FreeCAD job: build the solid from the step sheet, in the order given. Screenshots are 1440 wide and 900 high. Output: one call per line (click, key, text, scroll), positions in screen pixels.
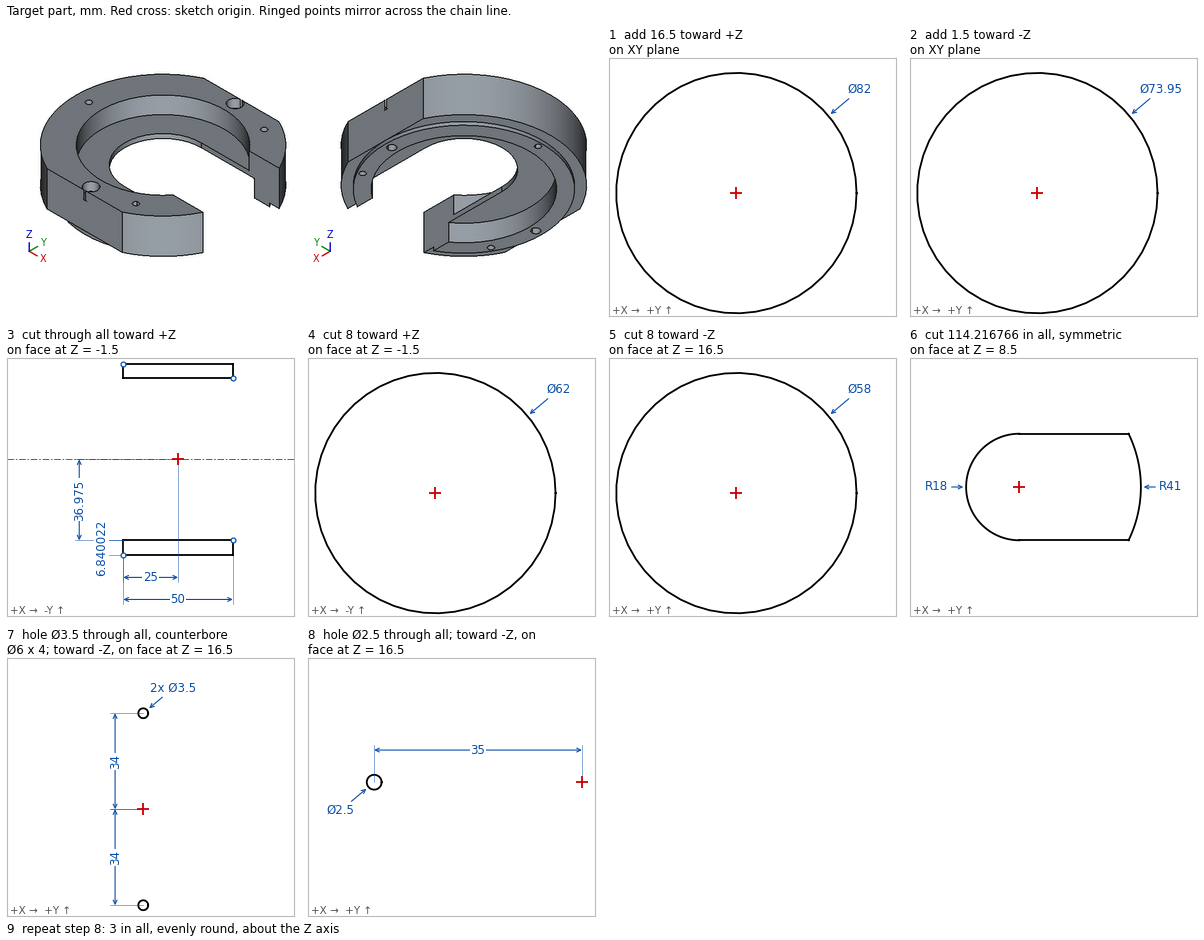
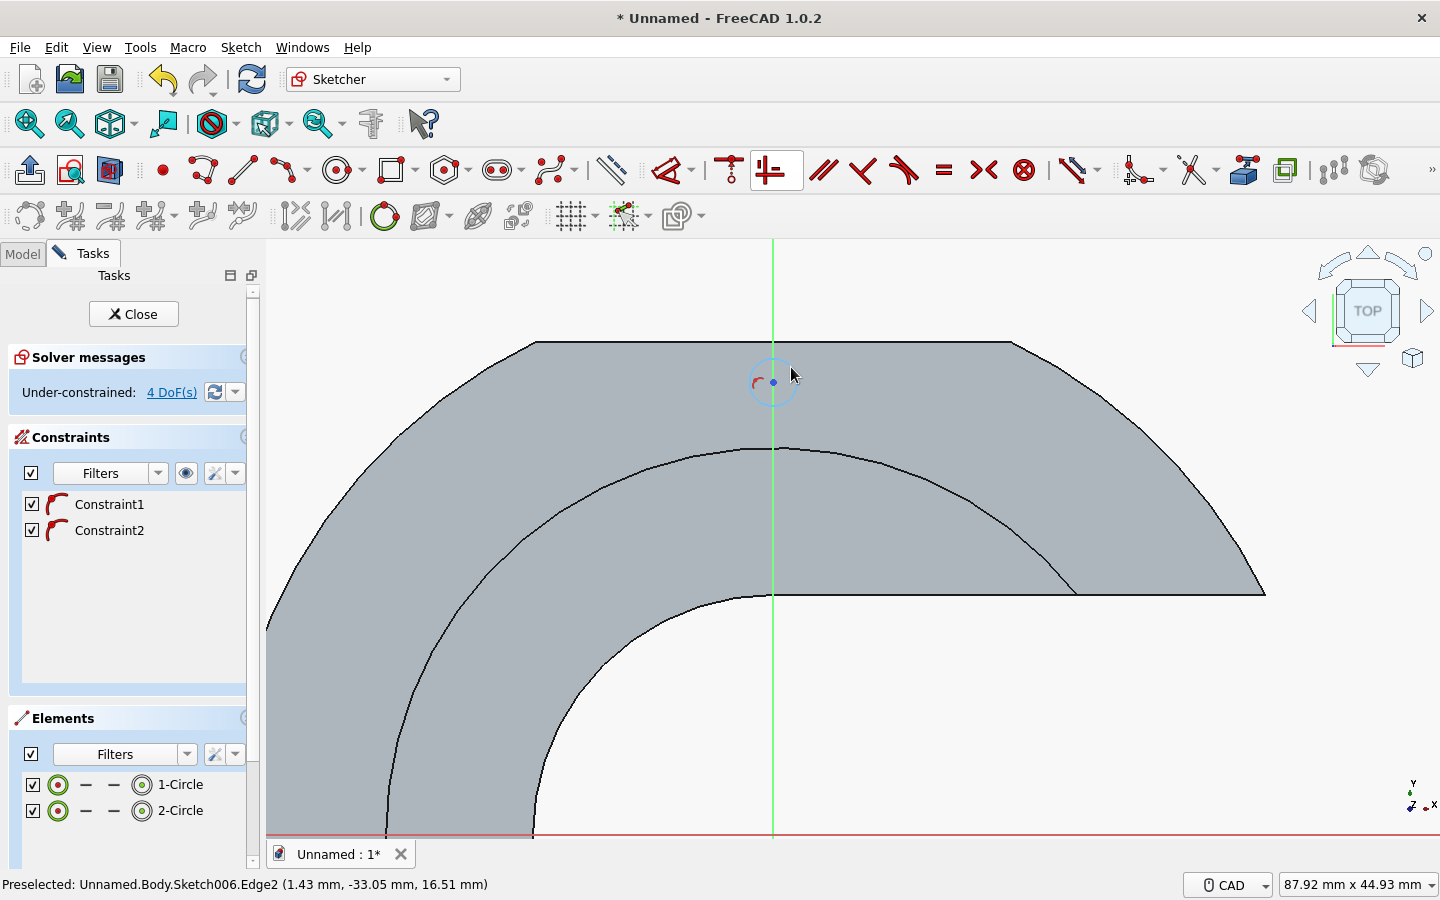
click(790, 366)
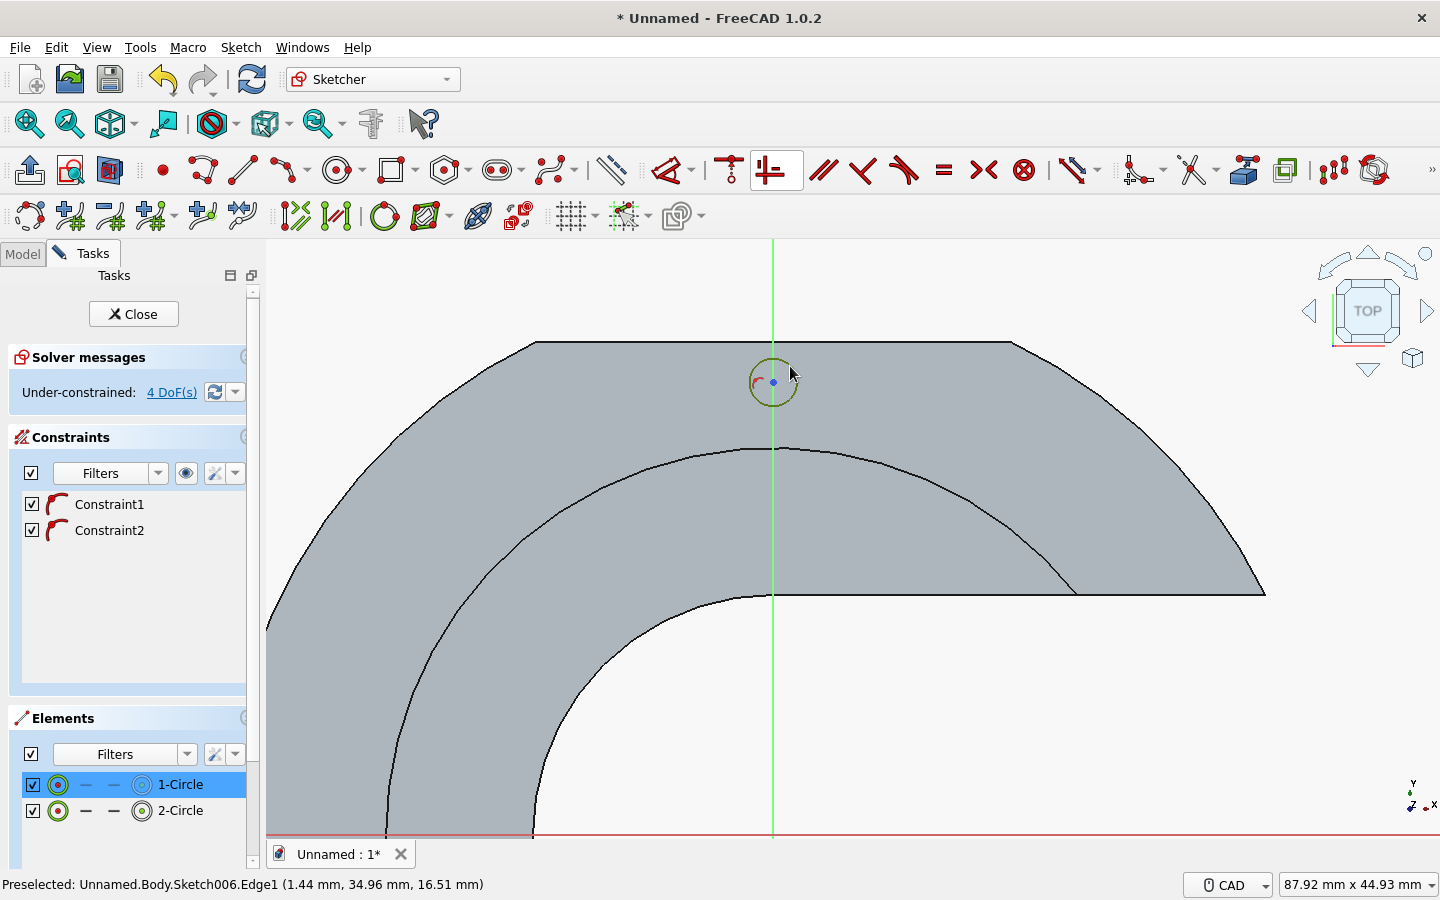
scroll(791, 367, down, 5)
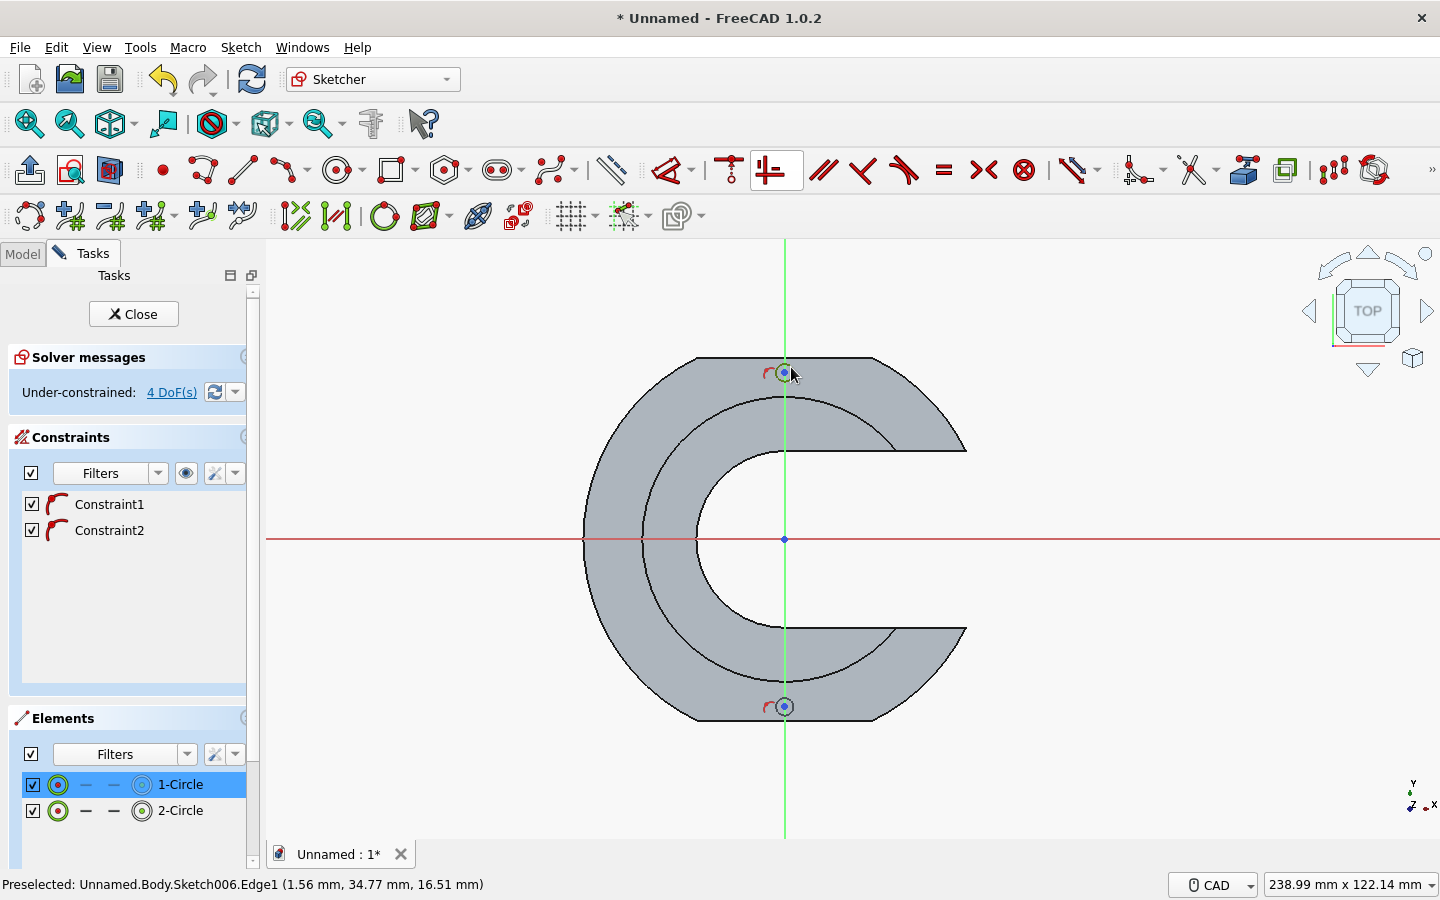
scroll(791, 701, up, 5)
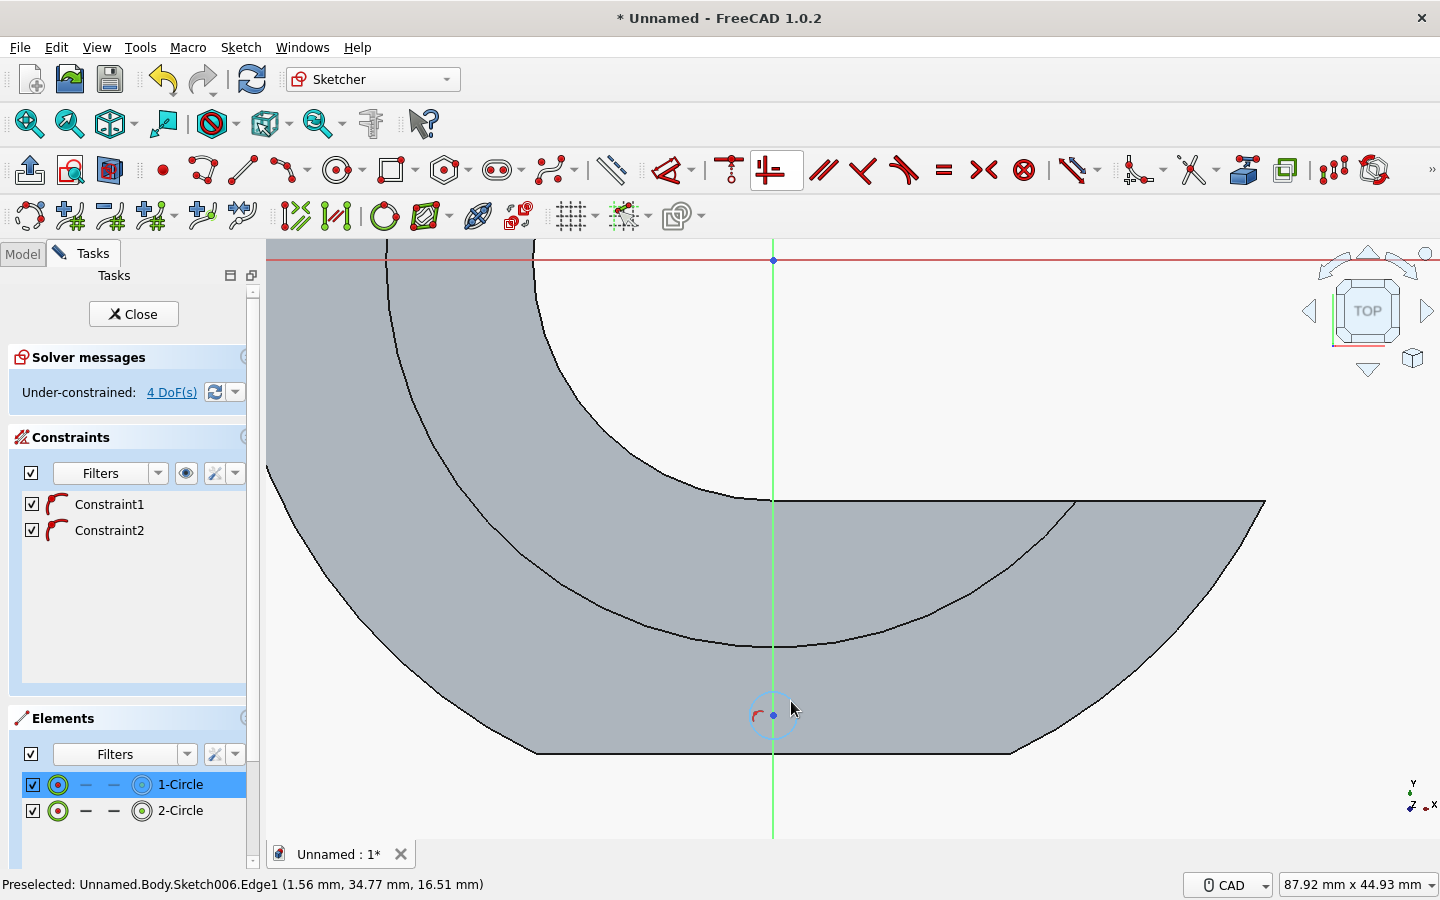
click(790, 699)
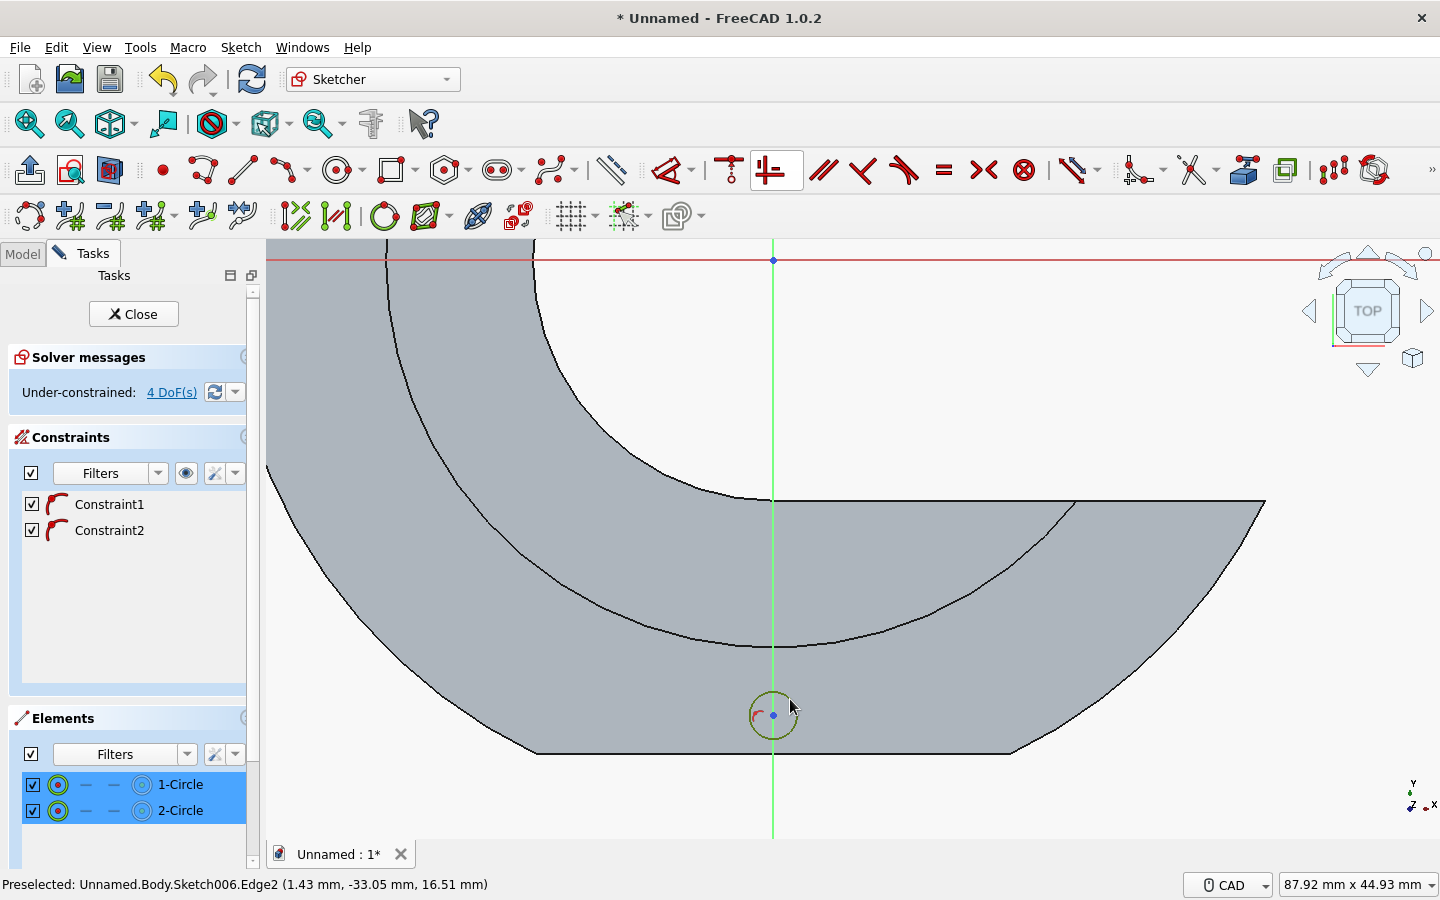
click(944, 170)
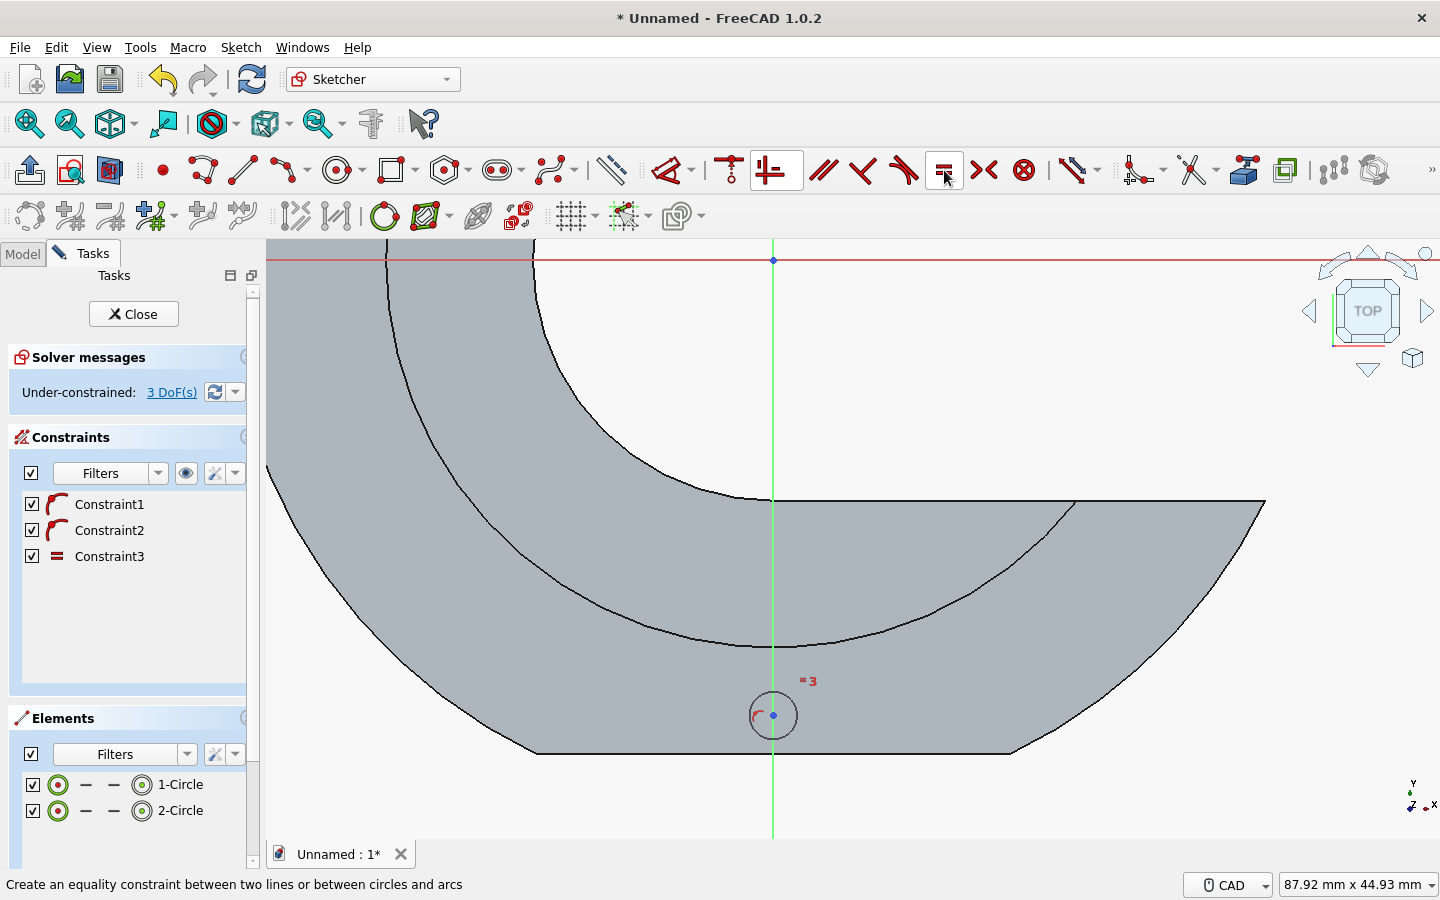
click(666, 170)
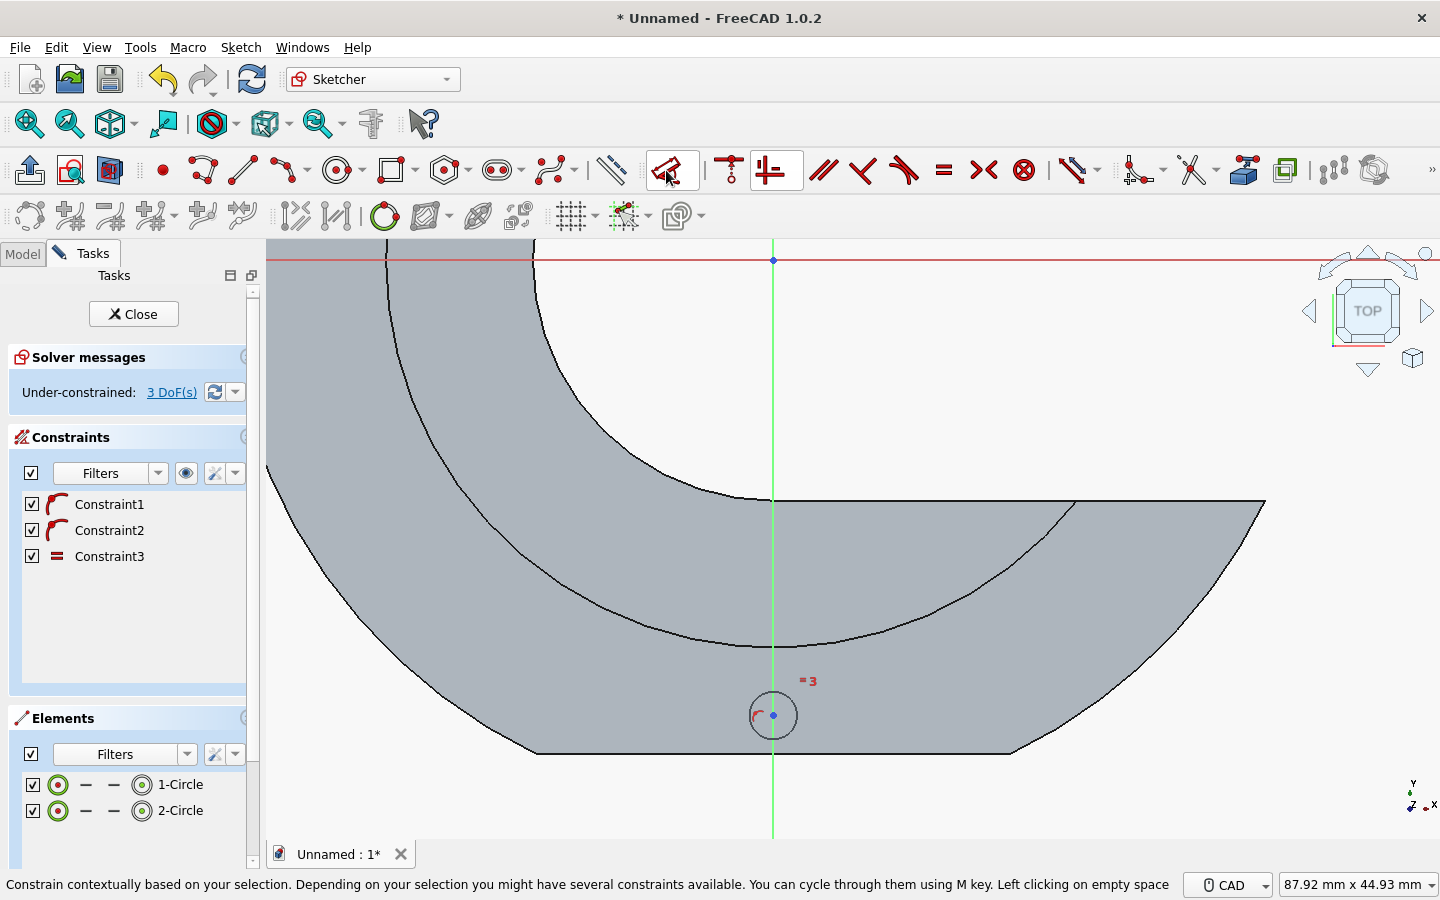
scroll(791, 701, down, 5)